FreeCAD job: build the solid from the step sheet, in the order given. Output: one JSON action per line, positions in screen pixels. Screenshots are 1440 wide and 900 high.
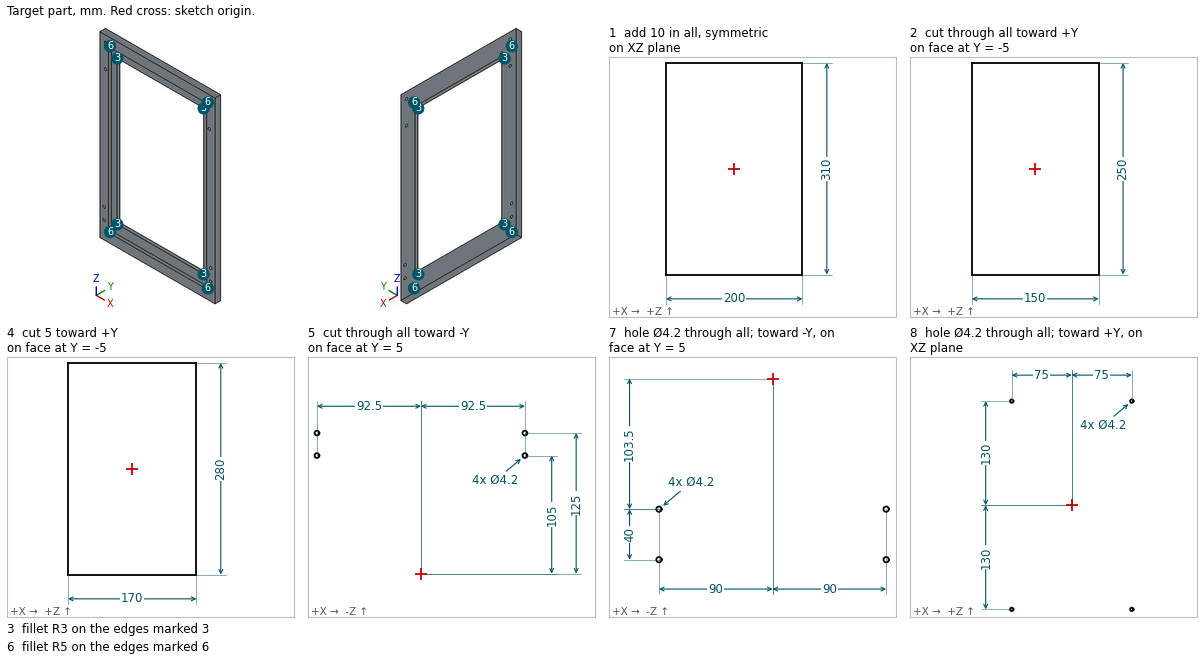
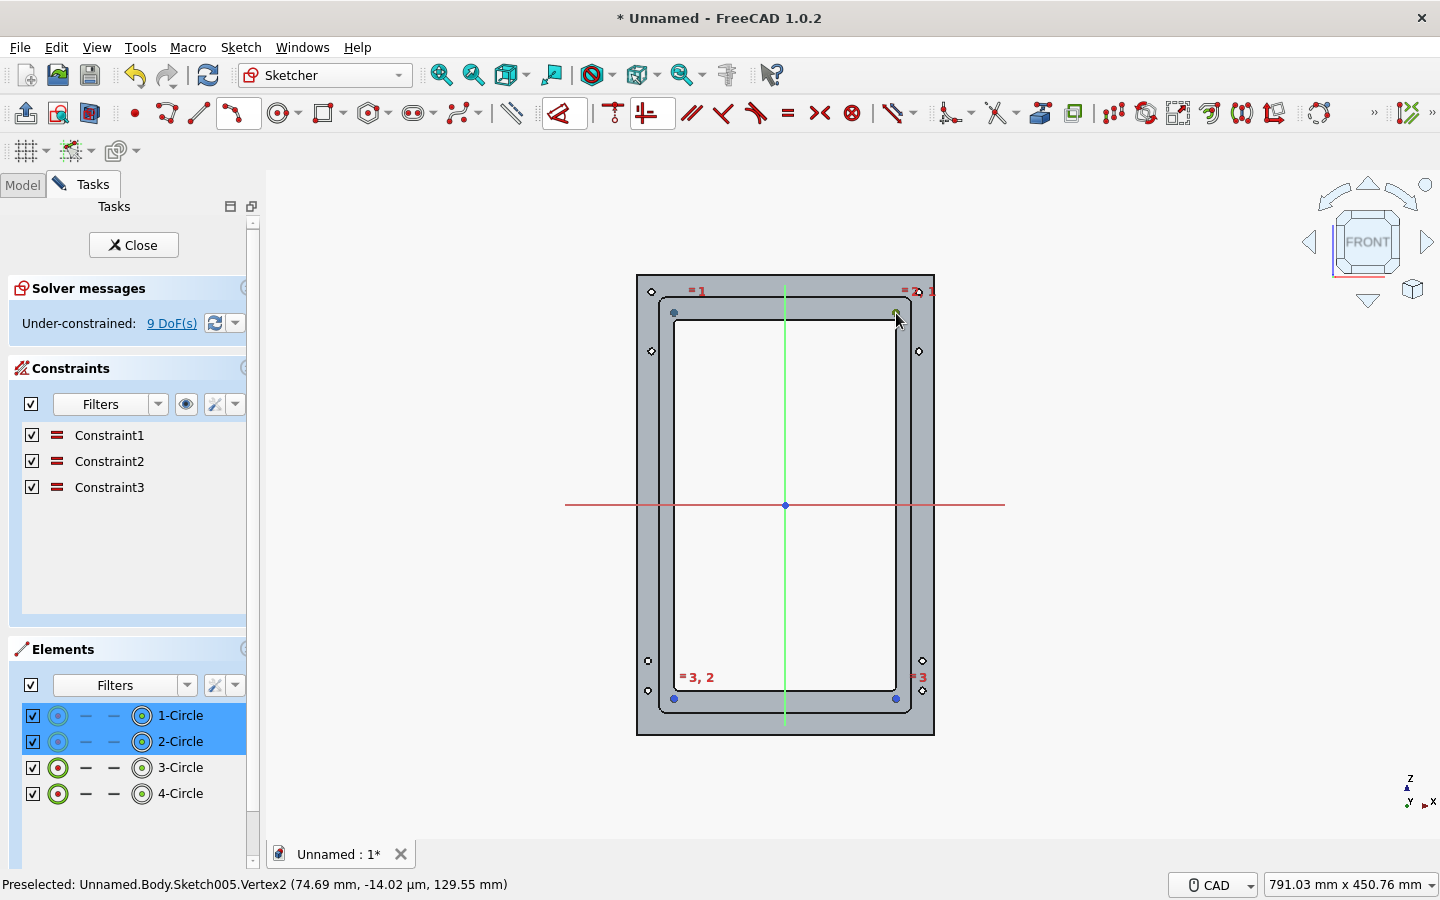
{"action": "key", "text": "h"}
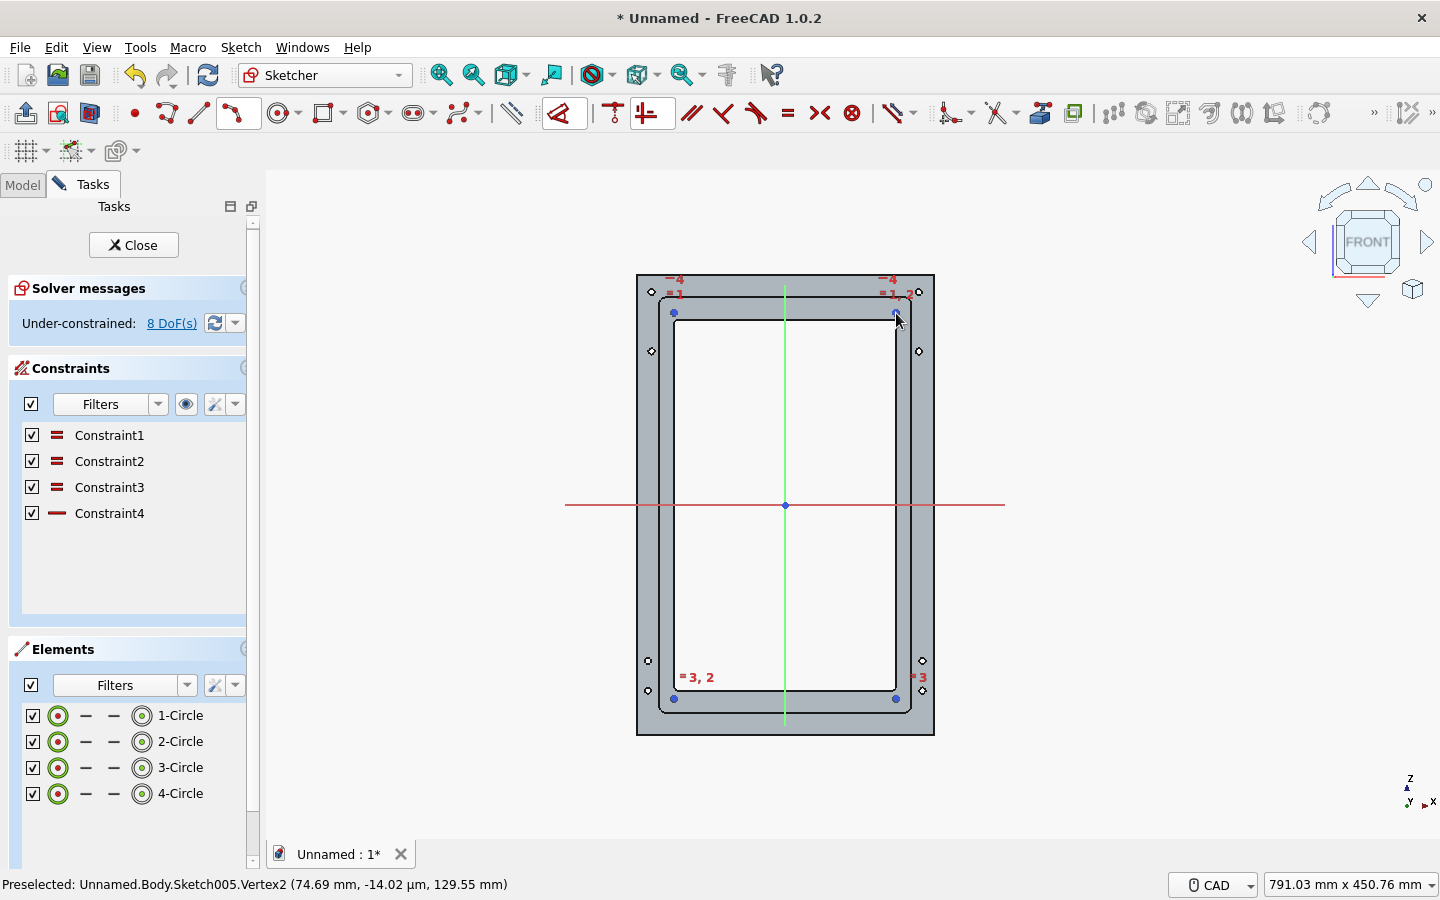
{"action": "left_click", "coordinate": [674, 313]}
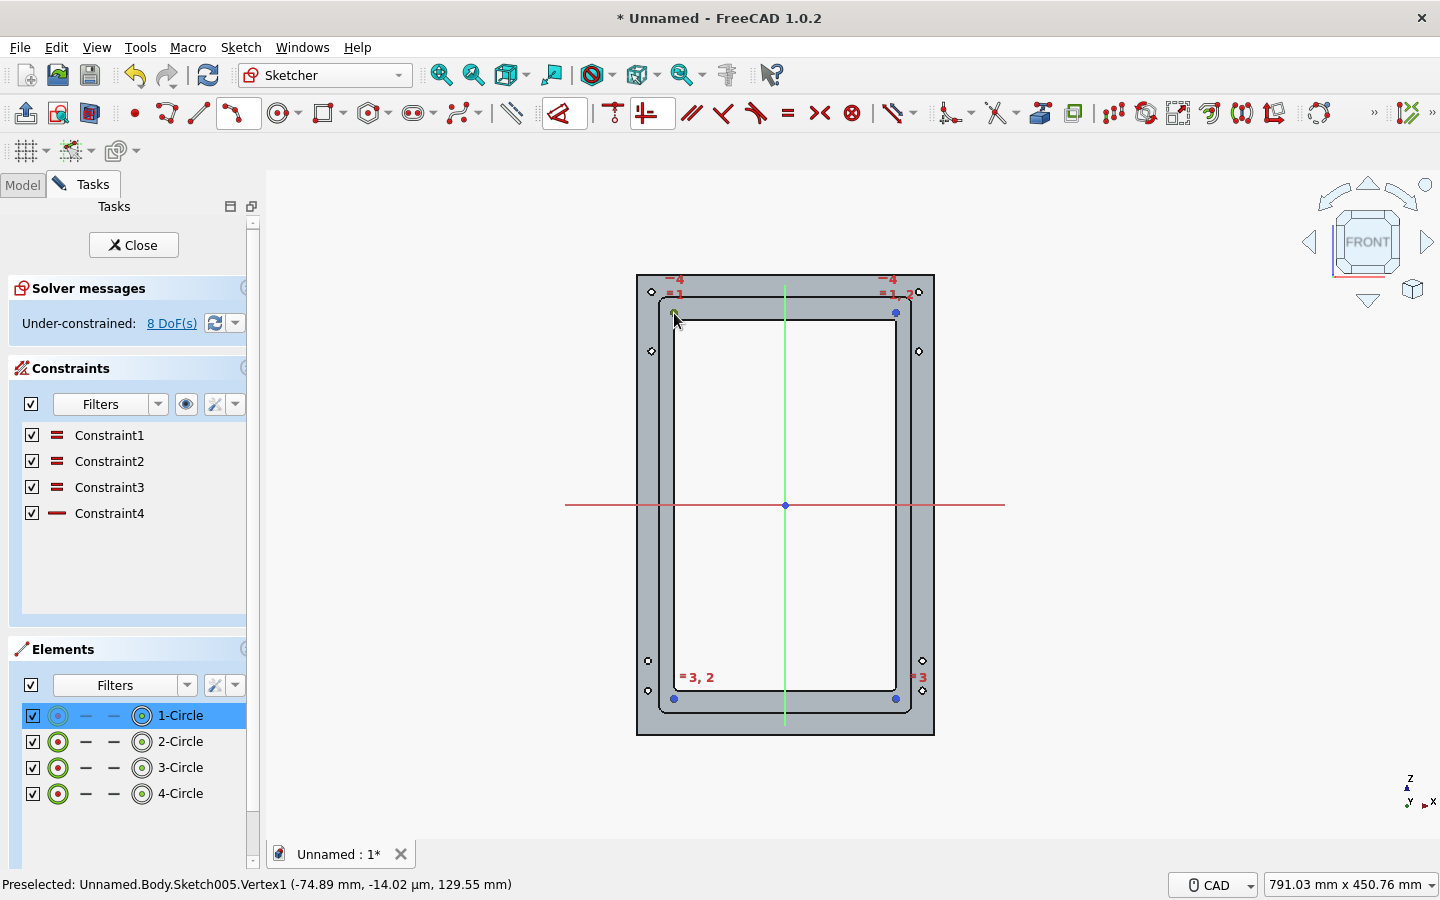
{"action": "left_click", "coordinate": [674, 699]}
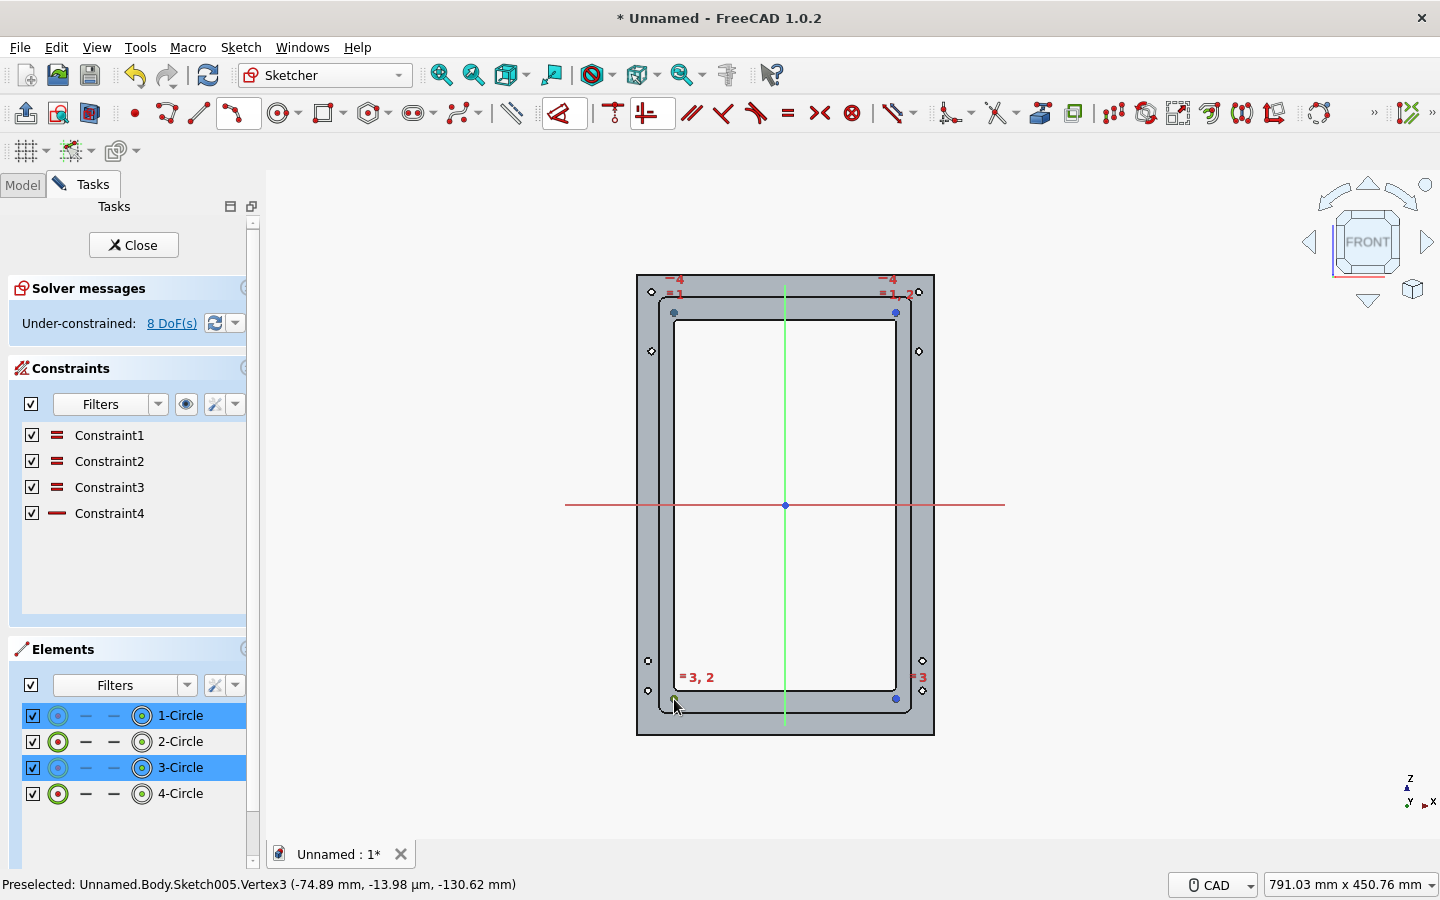
{"action": "key", "text": "v"}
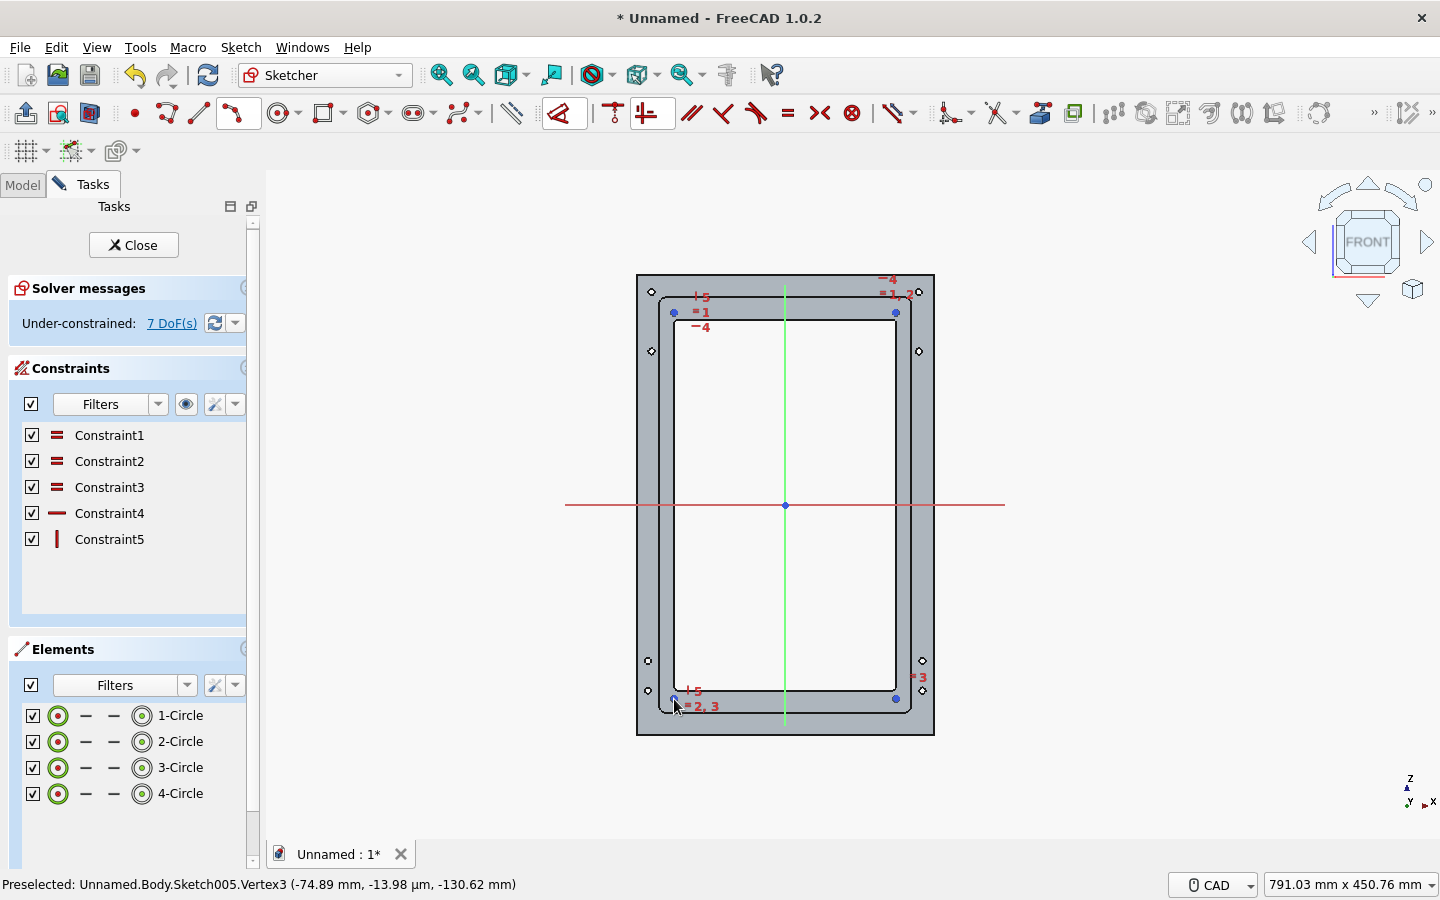
{"action": "left_click", "coordinate": [896, 313]}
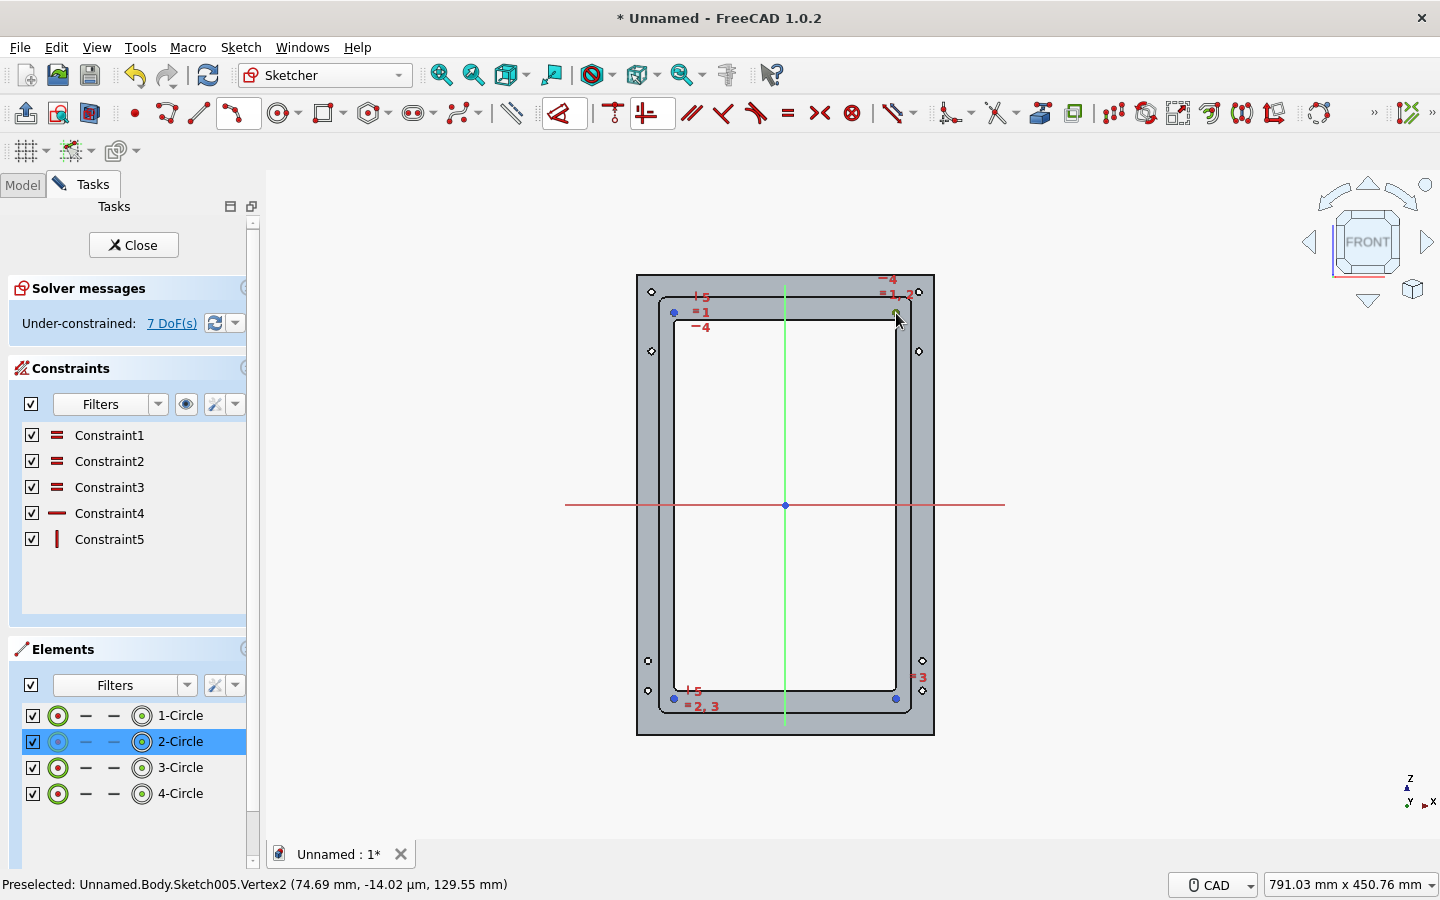
{"action": "left_click", "coordinate": [896, 699]}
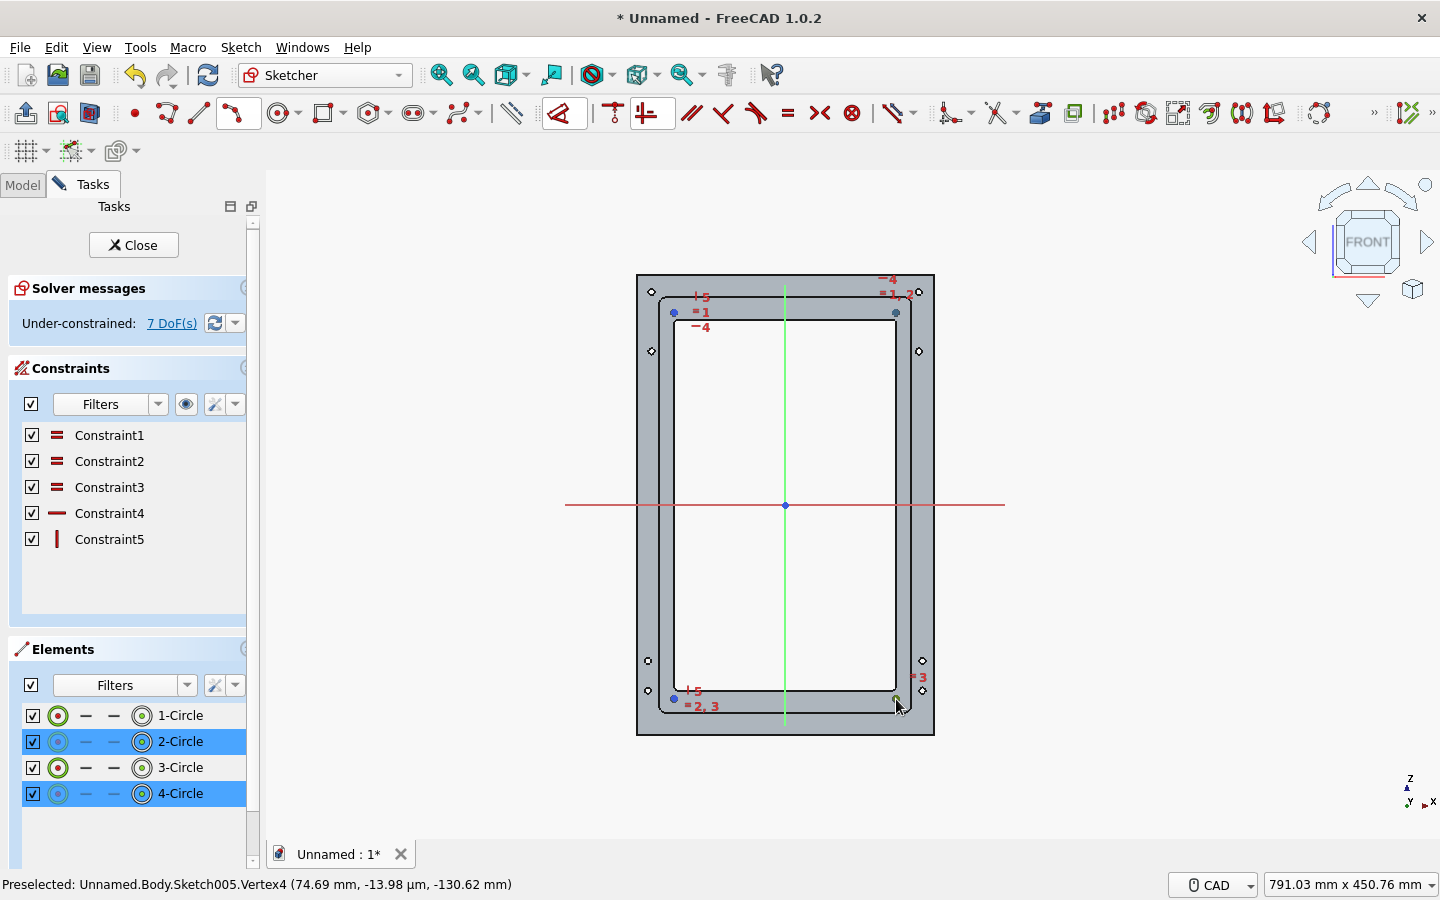
{"action": "key", "text": "v"}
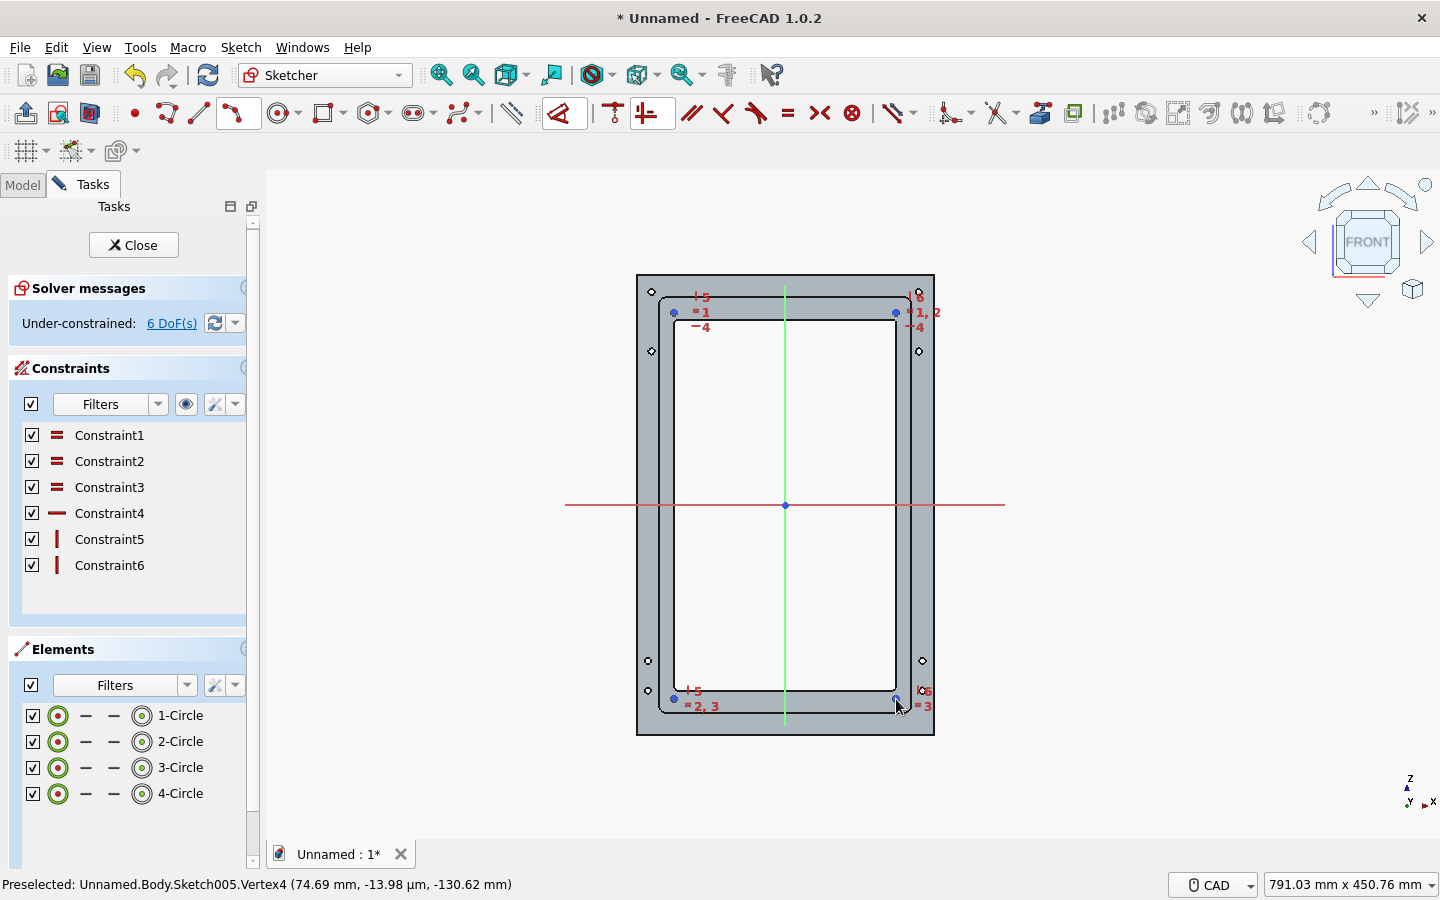
{"action": "left_click", "coordinate": [674, 699]}